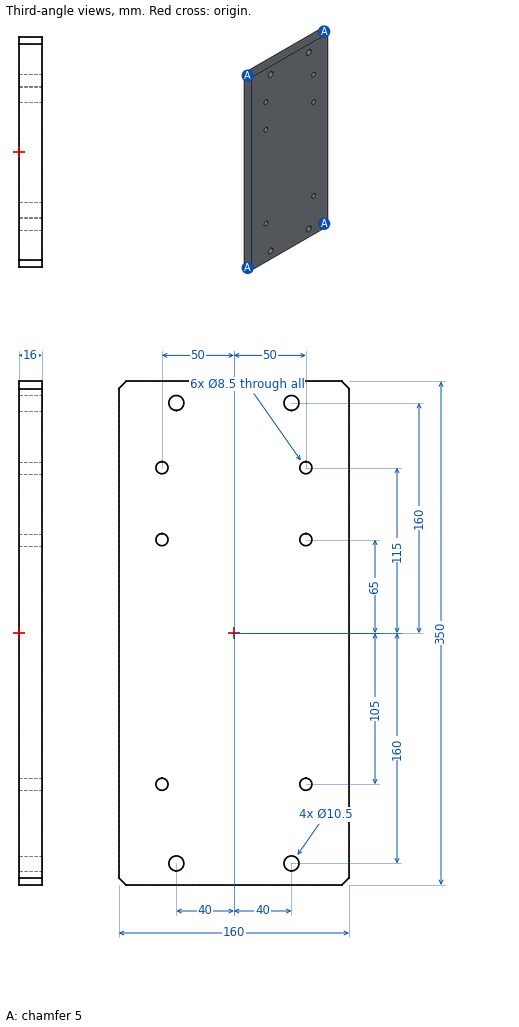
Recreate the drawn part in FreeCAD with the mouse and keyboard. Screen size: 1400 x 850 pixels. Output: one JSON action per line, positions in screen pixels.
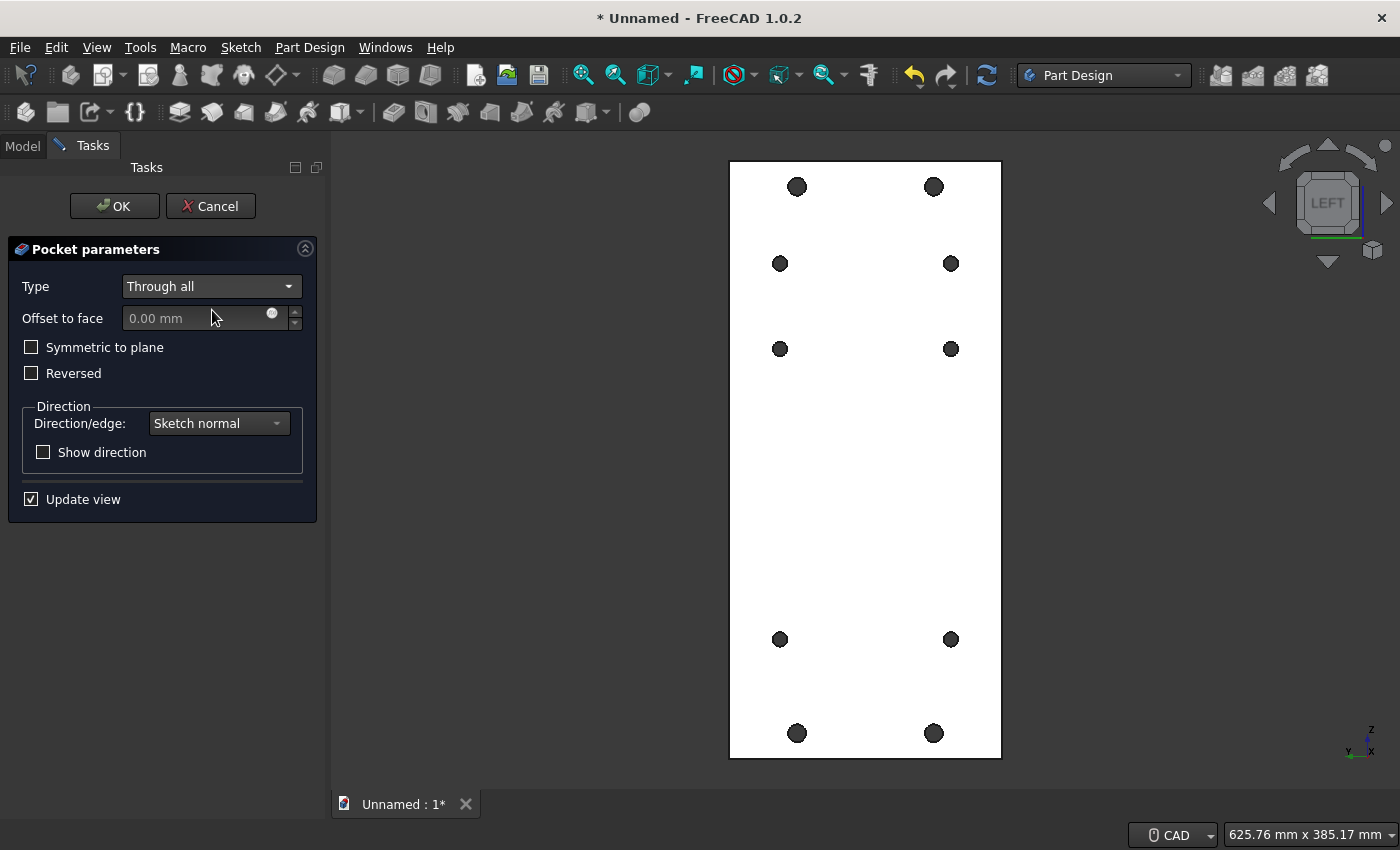
{"action": "left_click", "coordinate": [115, 206]}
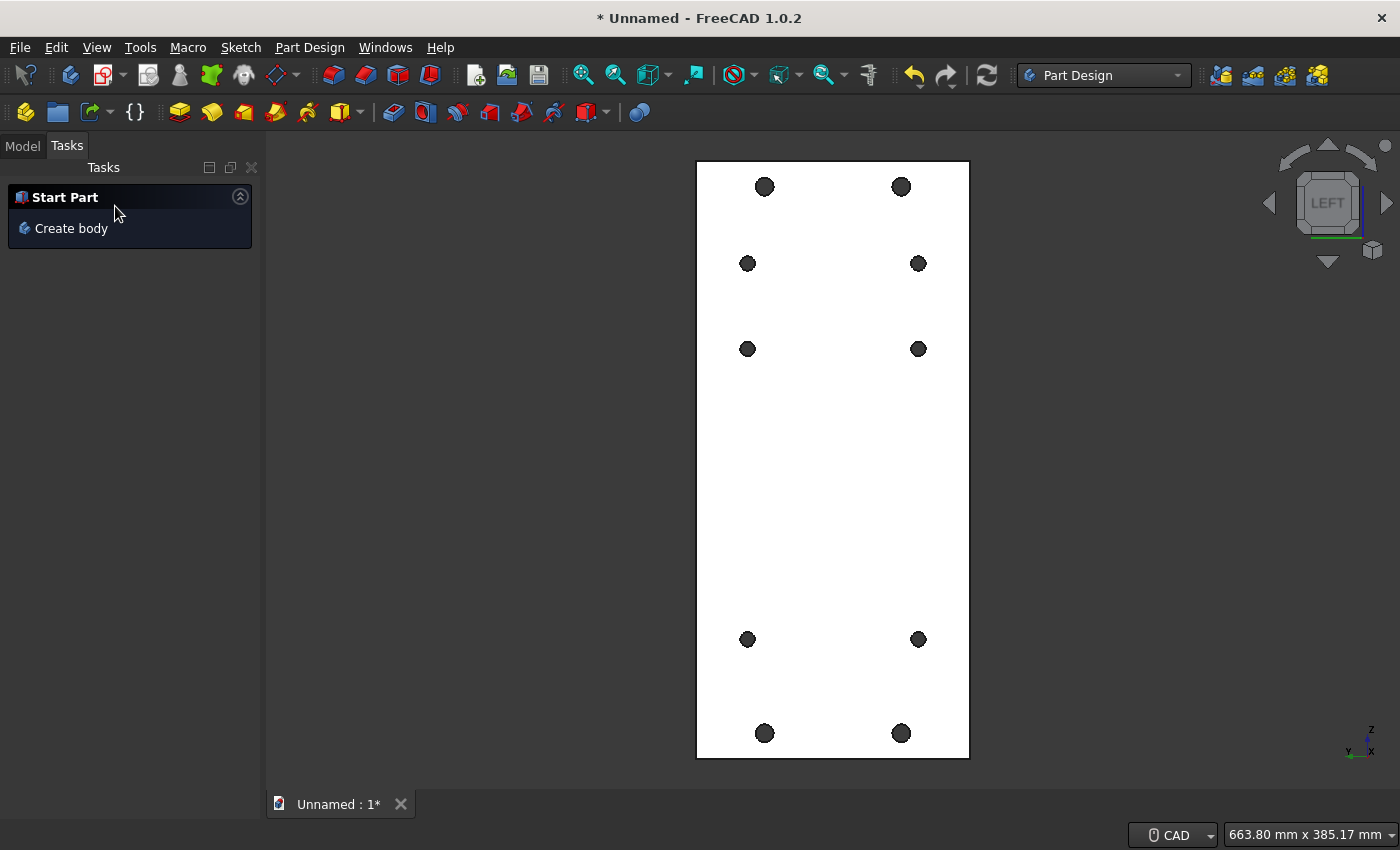
{"action": "key", "text": "0"}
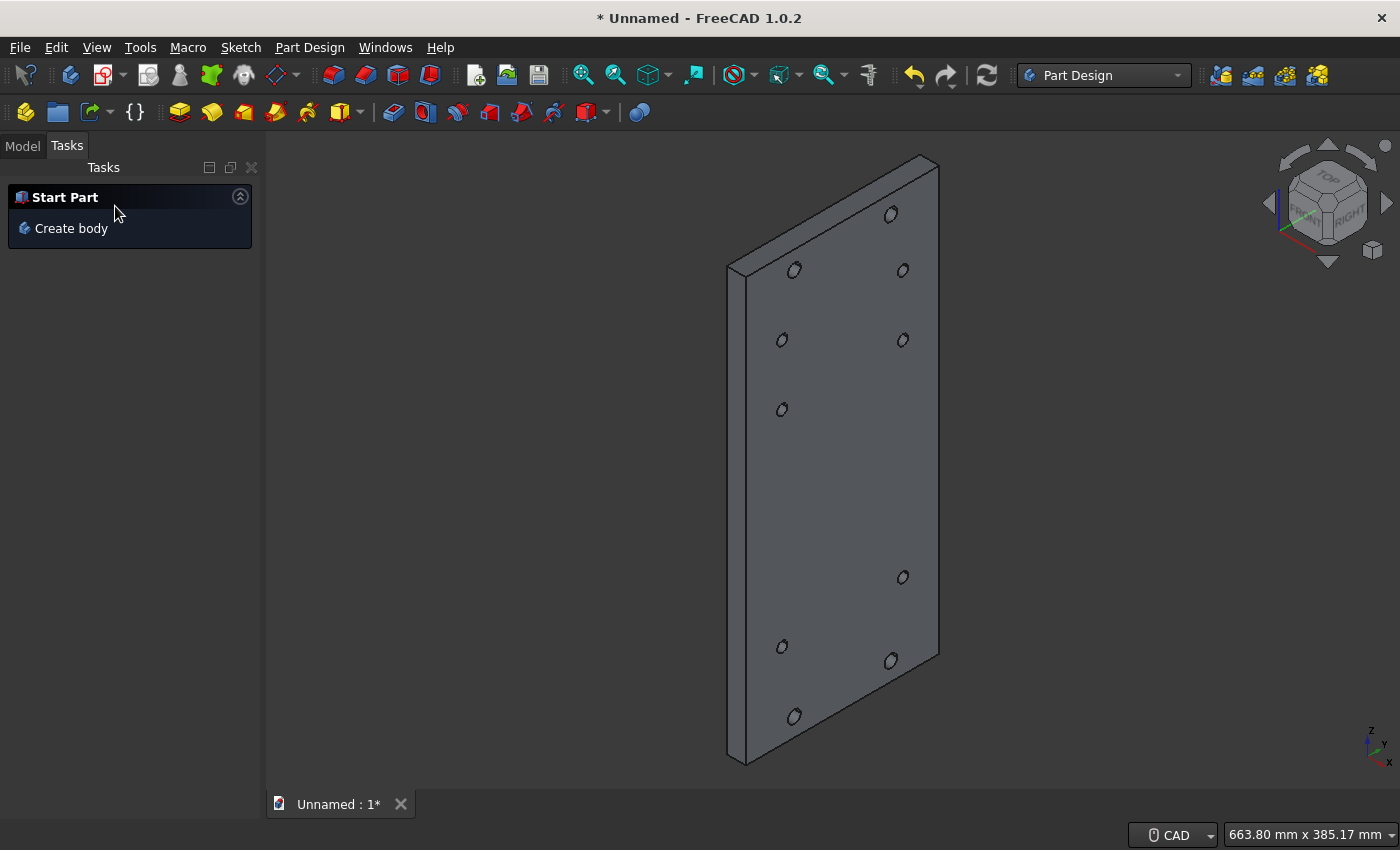
{"action": "left_click", "coordinate": [736, 271]}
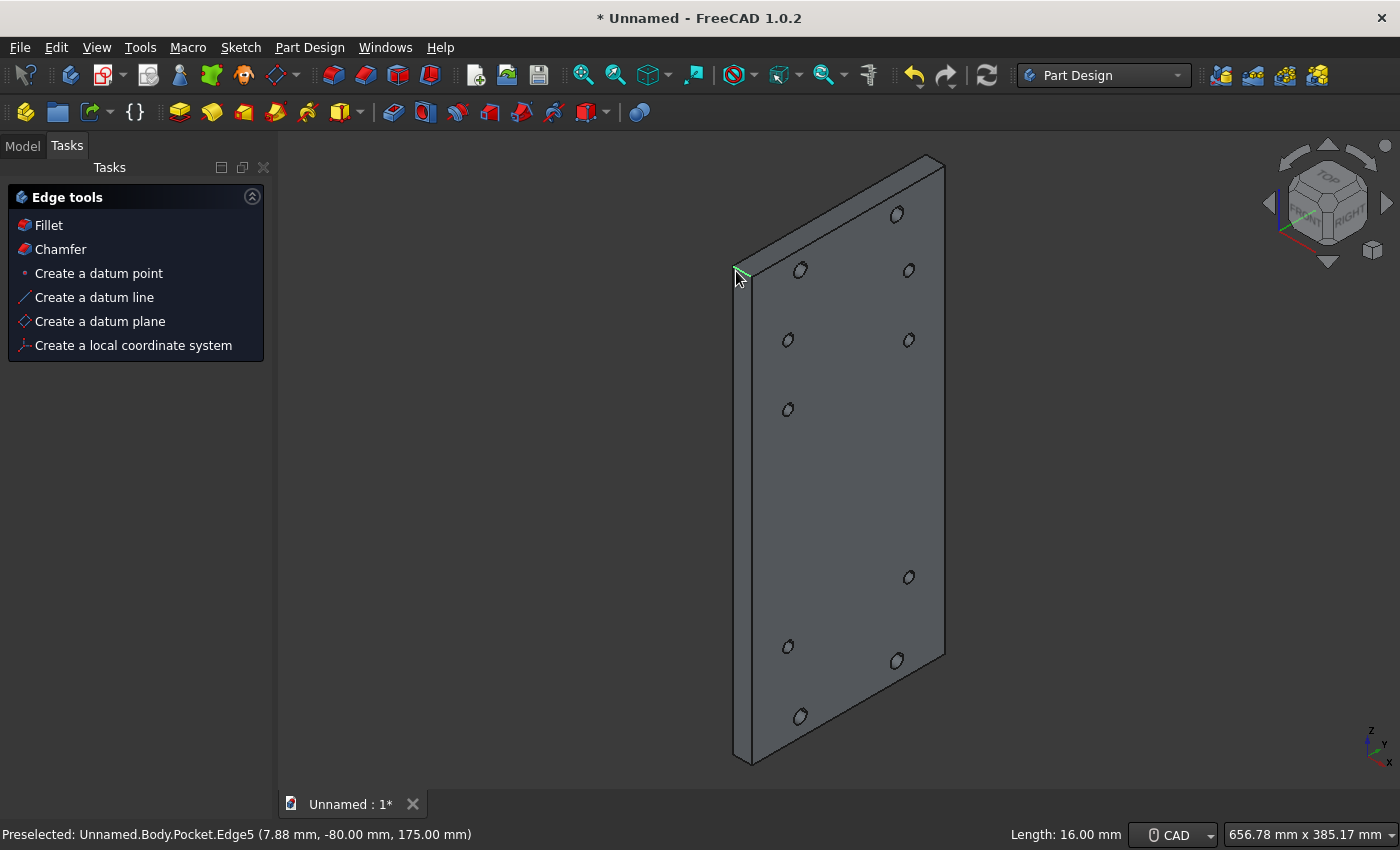
{"action": "key", "text": "2"}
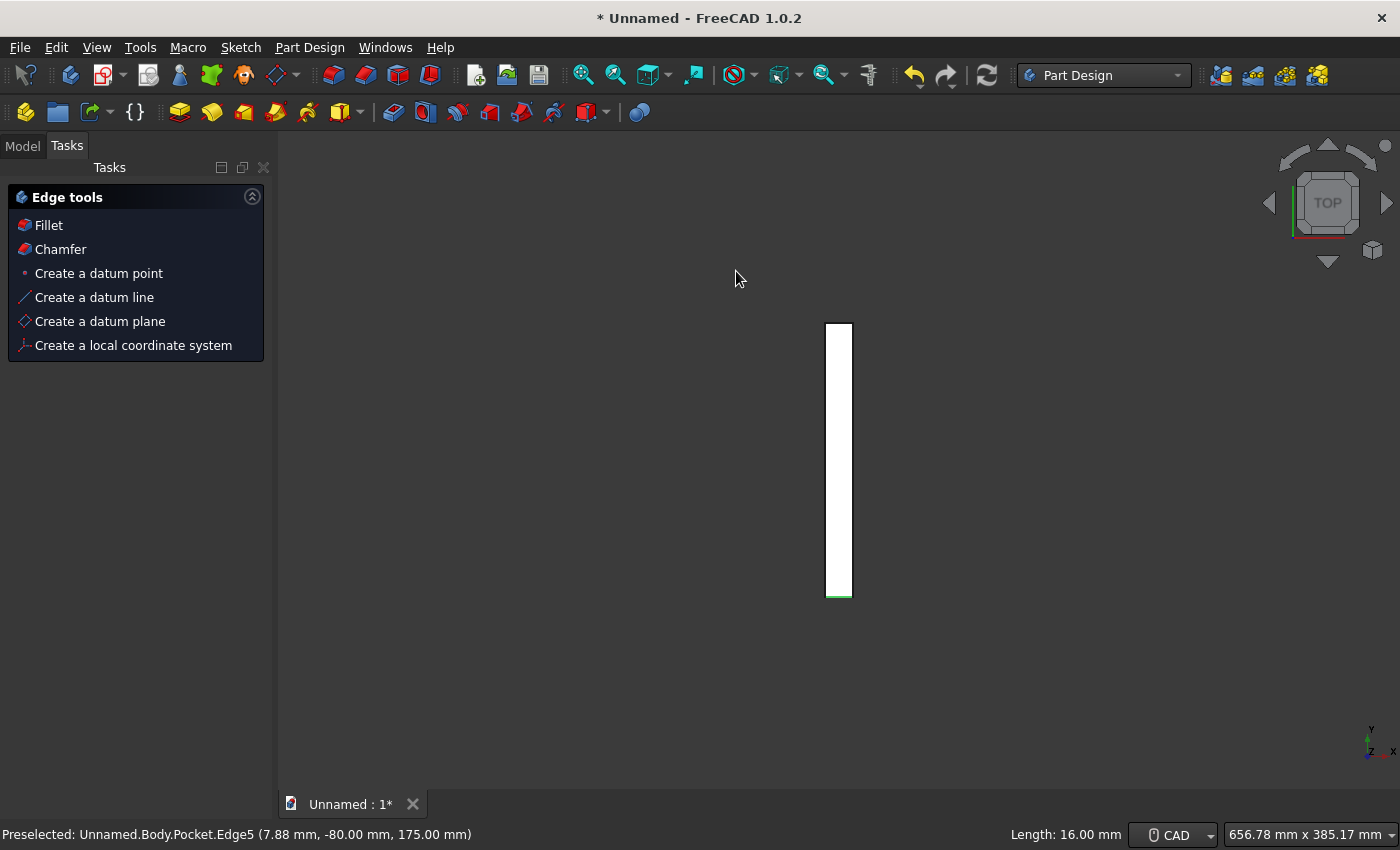
{"action": "left_click", "coordinate": [584, 76]}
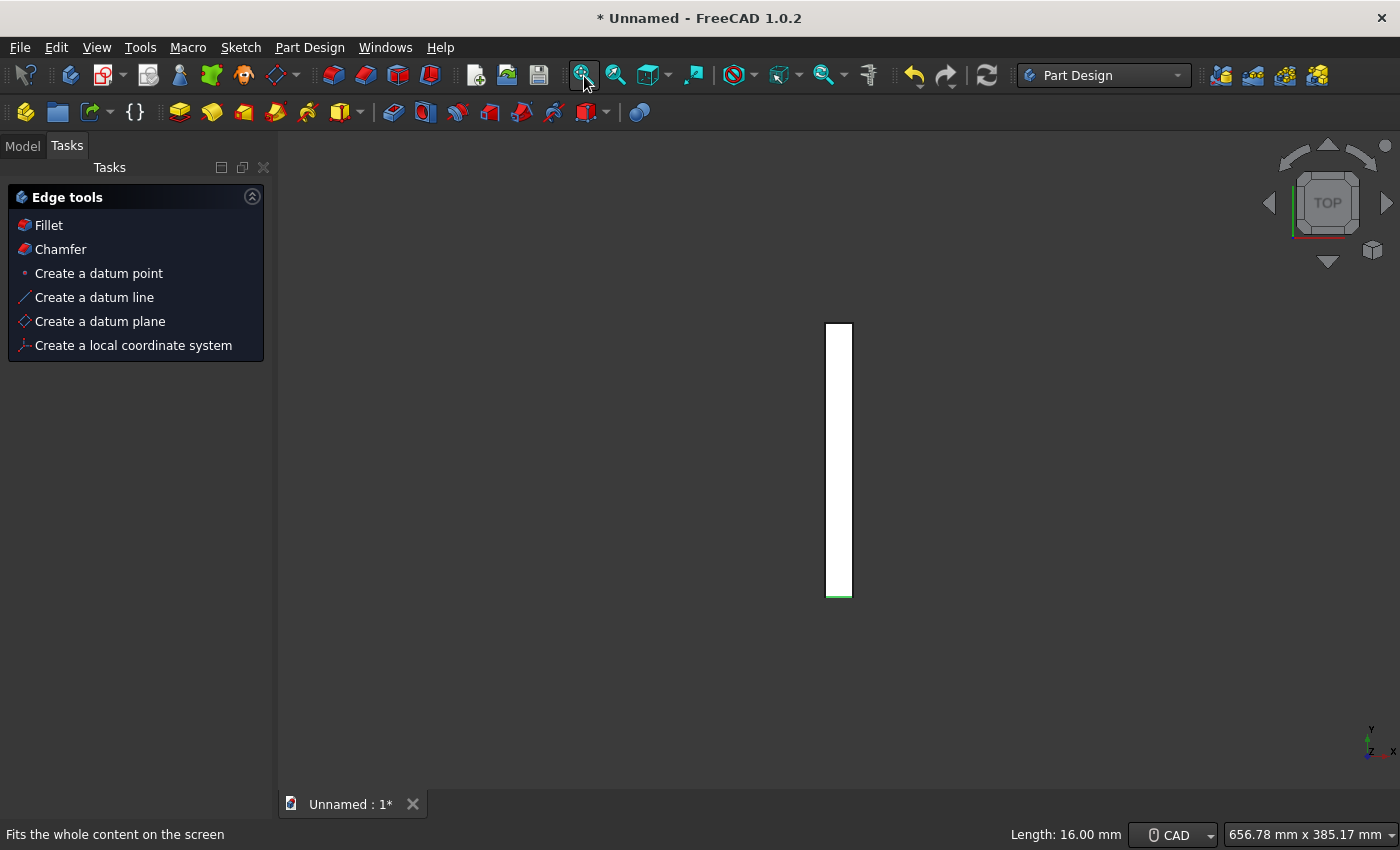
{"action": "left_click", "coordinate": [839, 322], "text": "ctrl"}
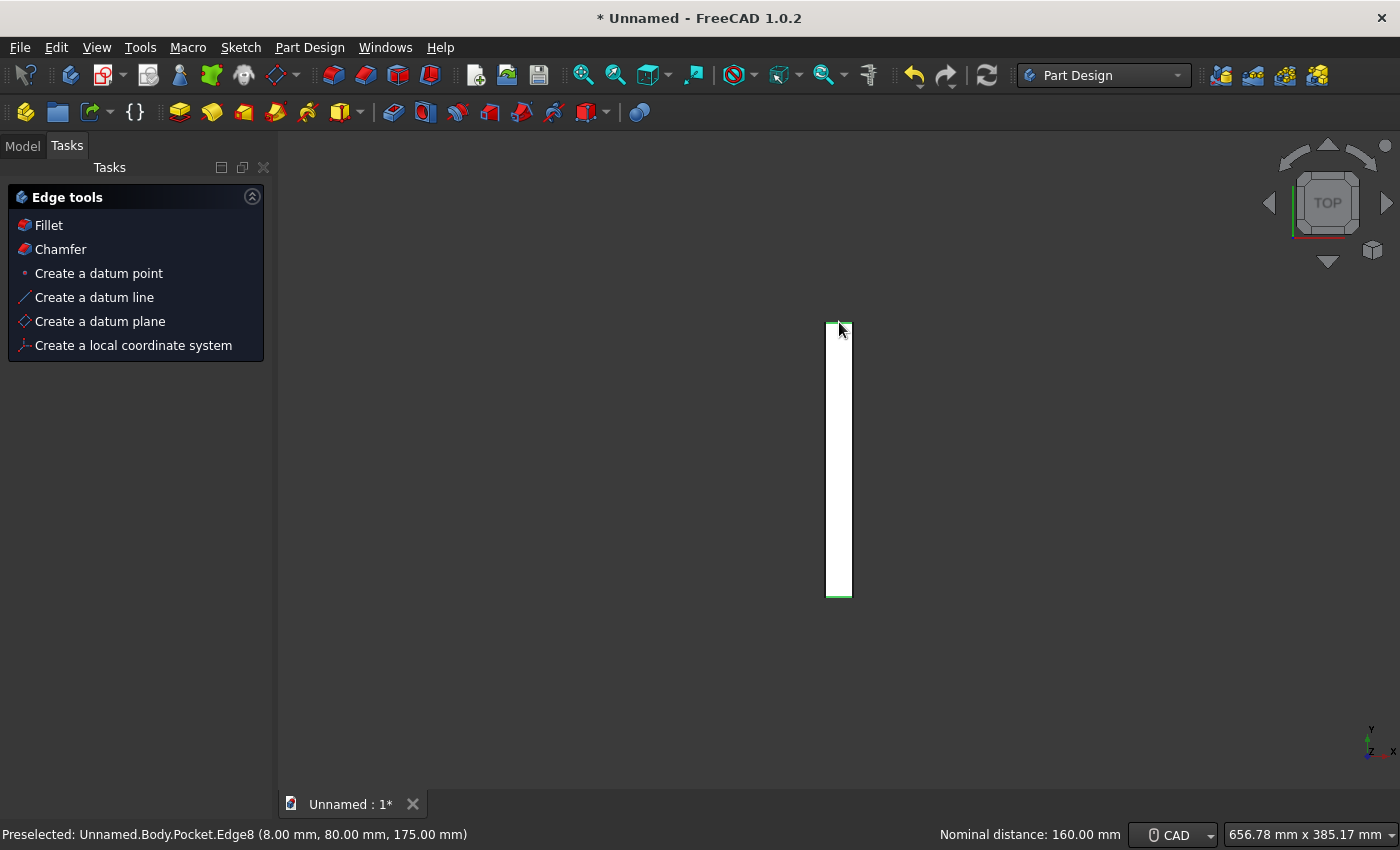
{"action": "key", "text": "1"}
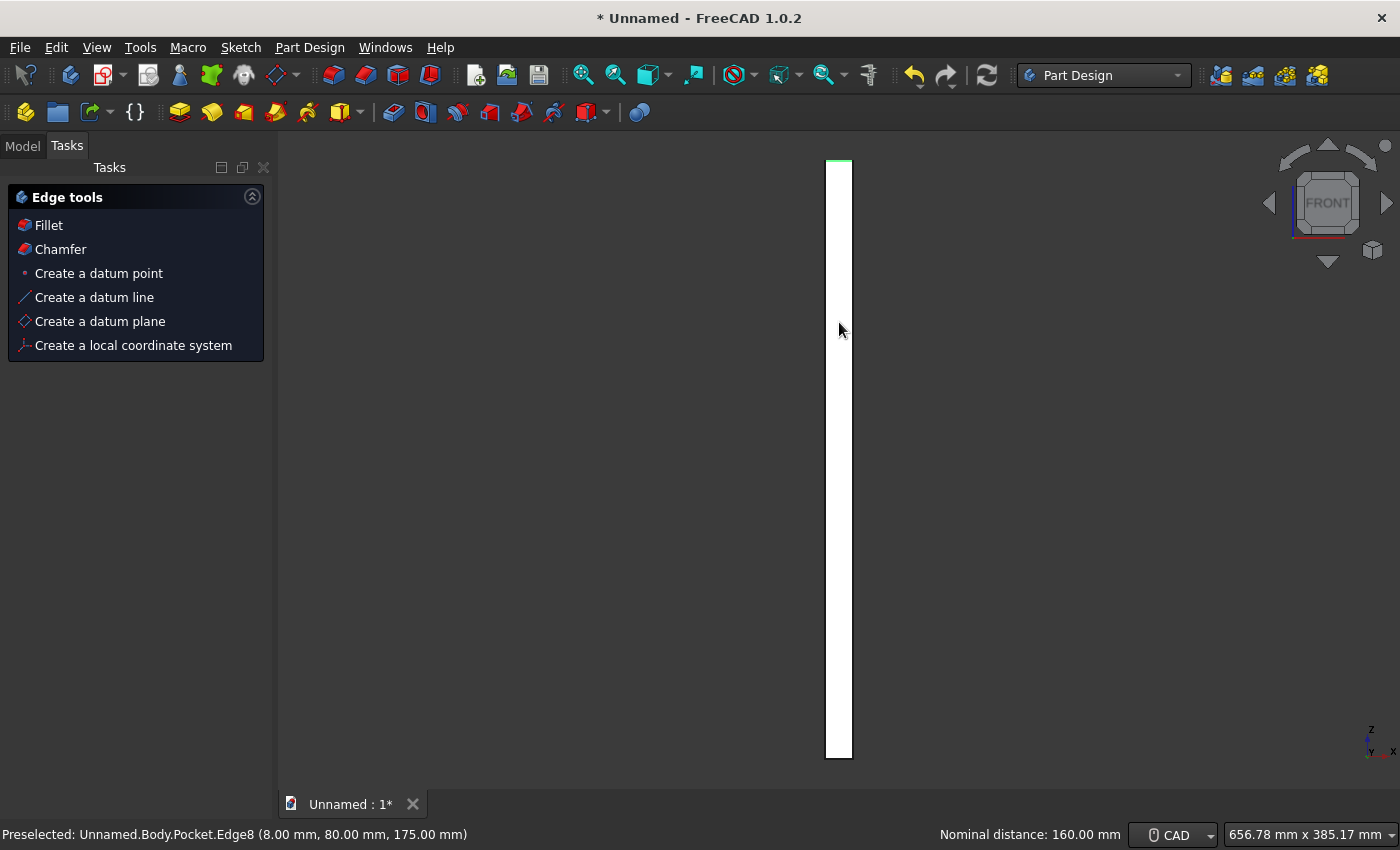
{"action": "left_click", "coordinate": [839, 758], "text": "ctrl"}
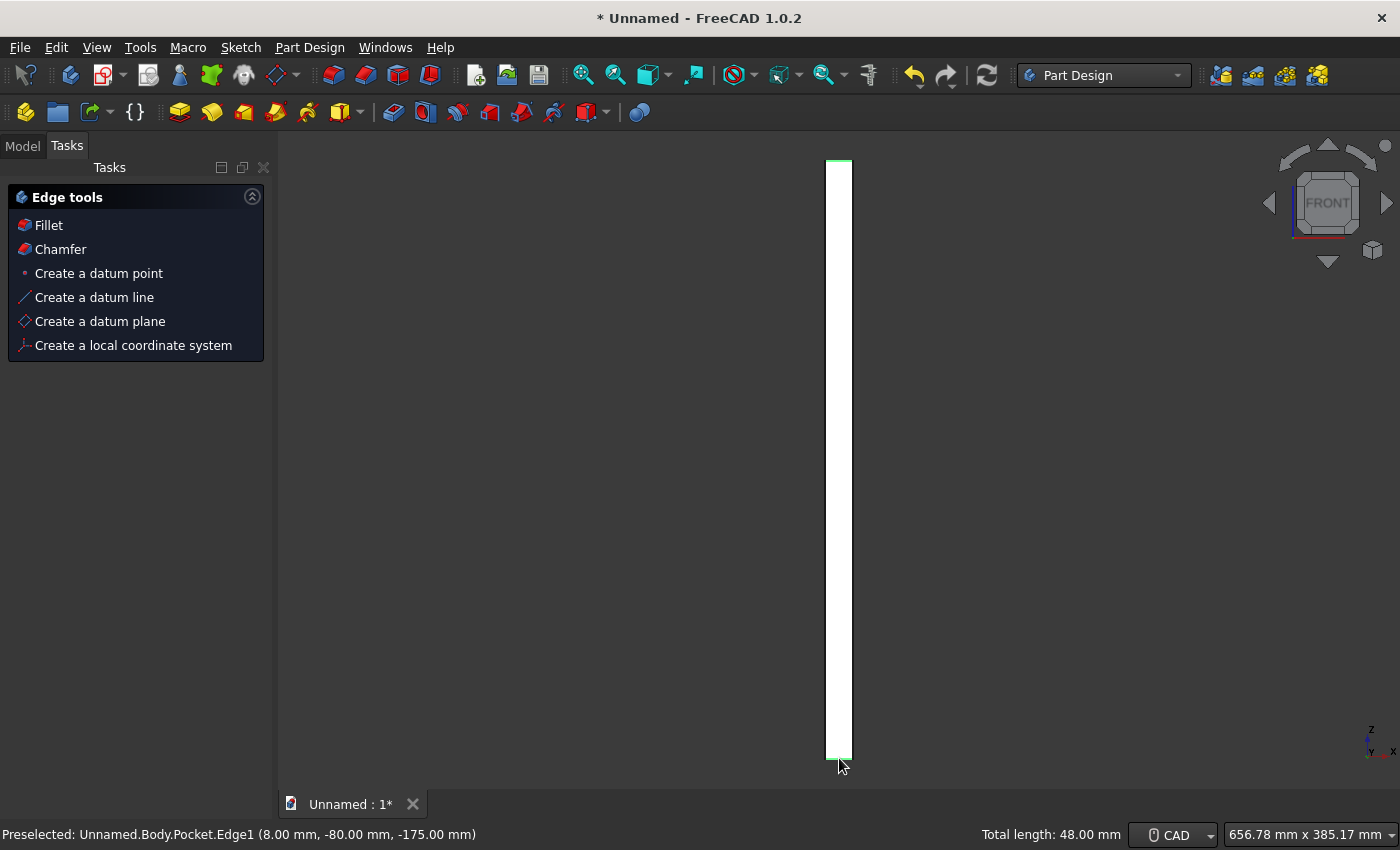
{"action": "key", "text": "3"}